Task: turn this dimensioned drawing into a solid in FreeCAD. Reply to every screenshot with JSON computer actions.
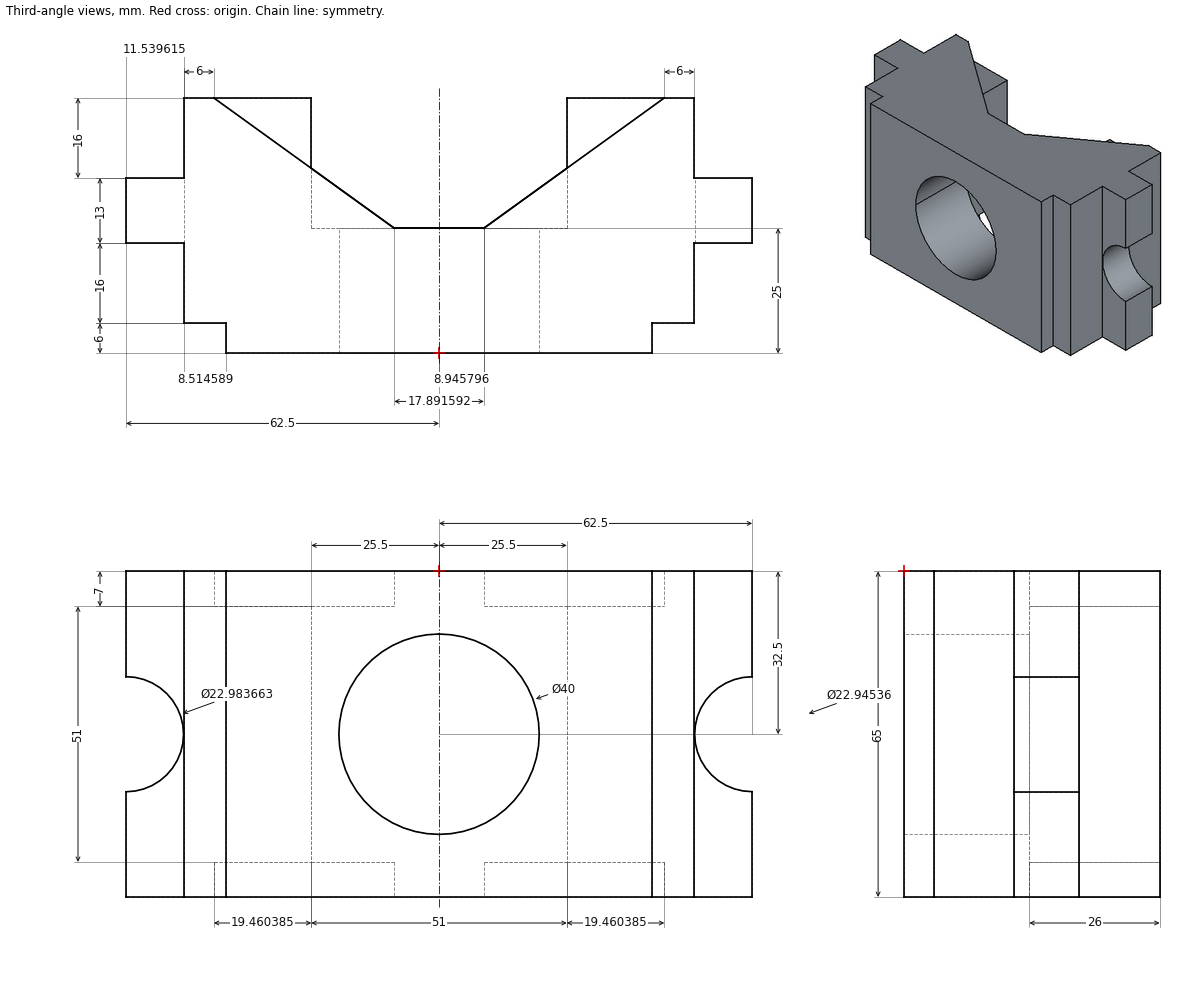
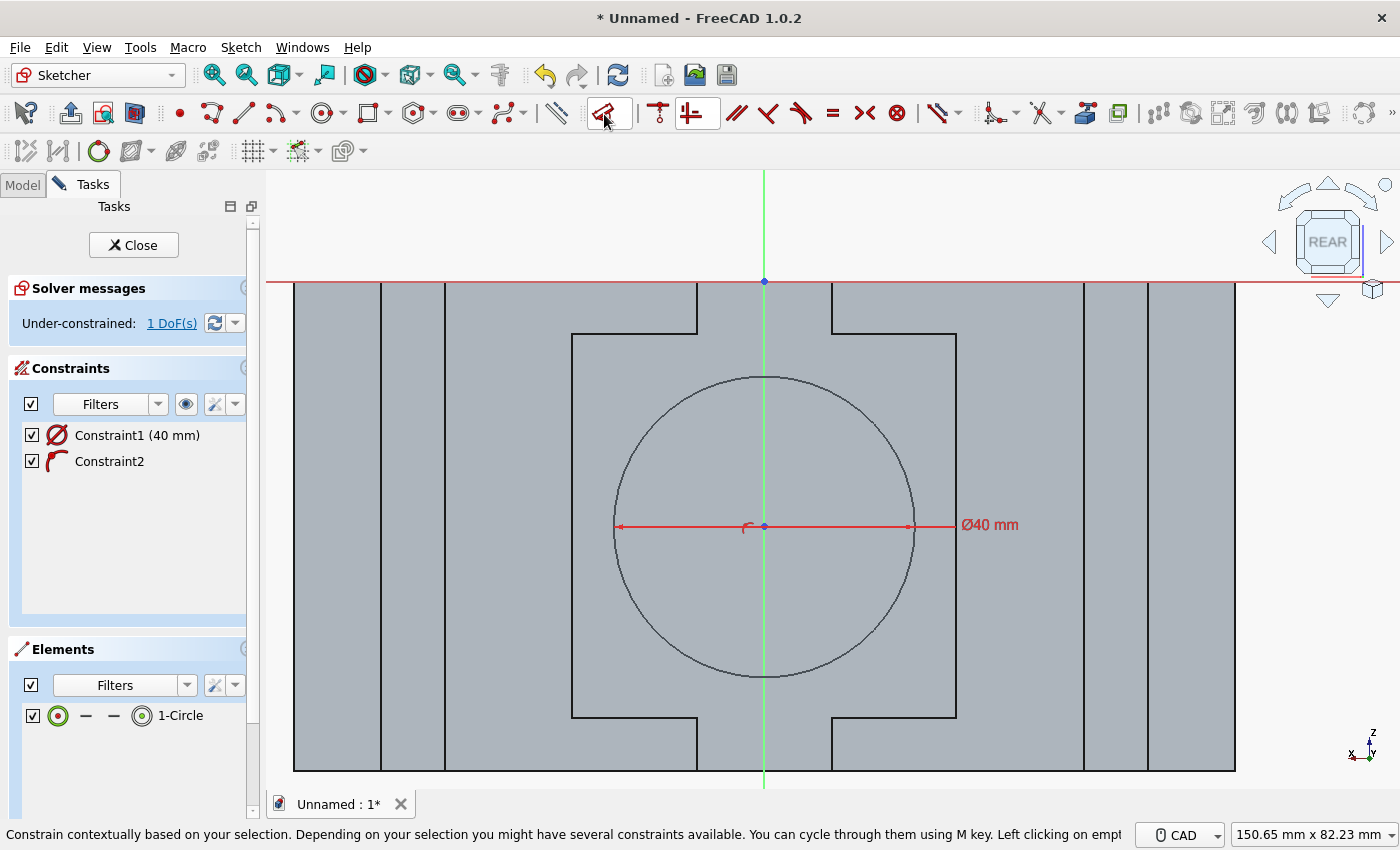
{"action": "left_click", "coordinate": [764, 527]}
{"action": "left_click", "coordinate": [798, 404]}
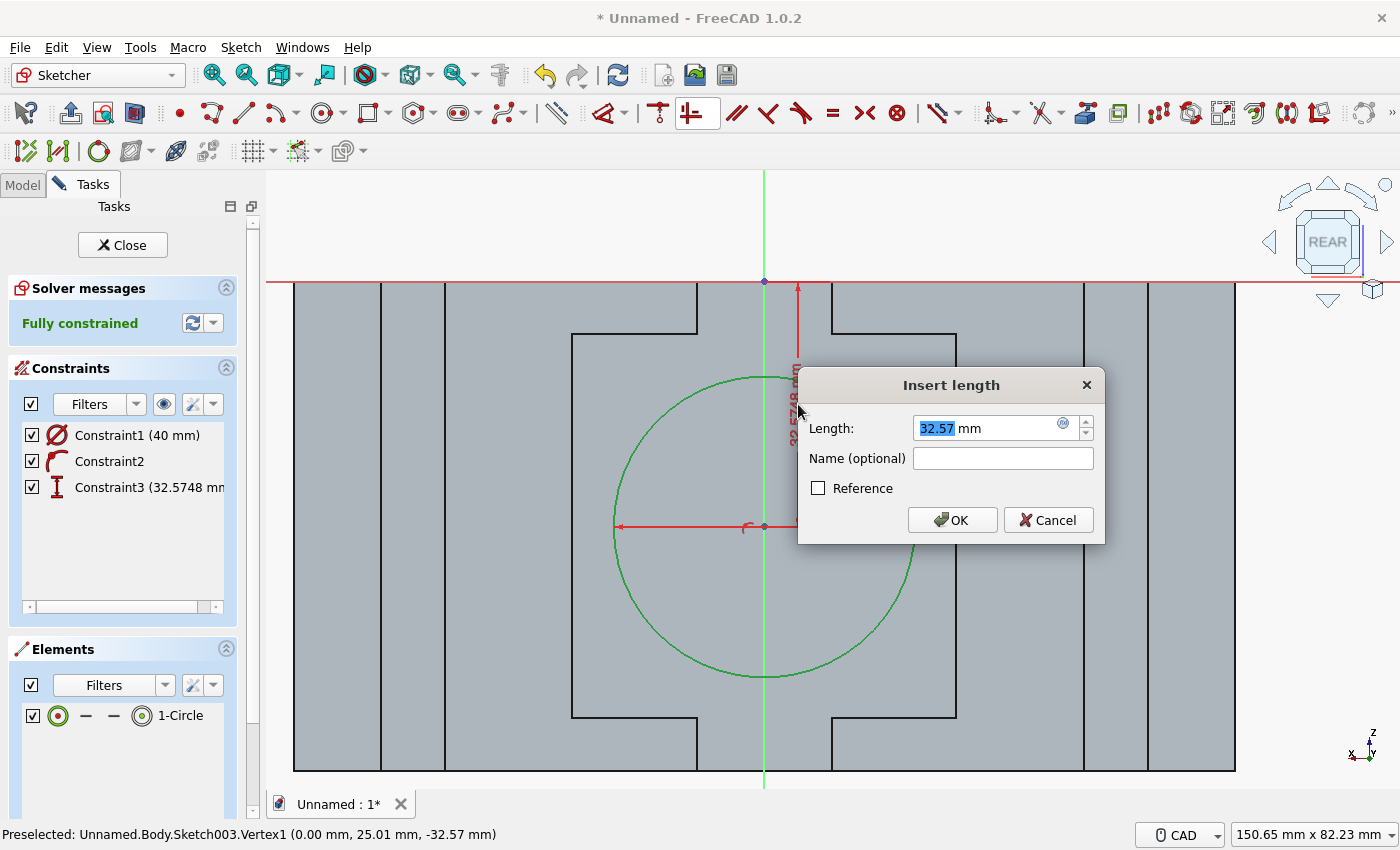
{"action": "type", "text": "32.5"}
{"action": "key", "text": "Return"}
{"action": "key", "text": "Escape"}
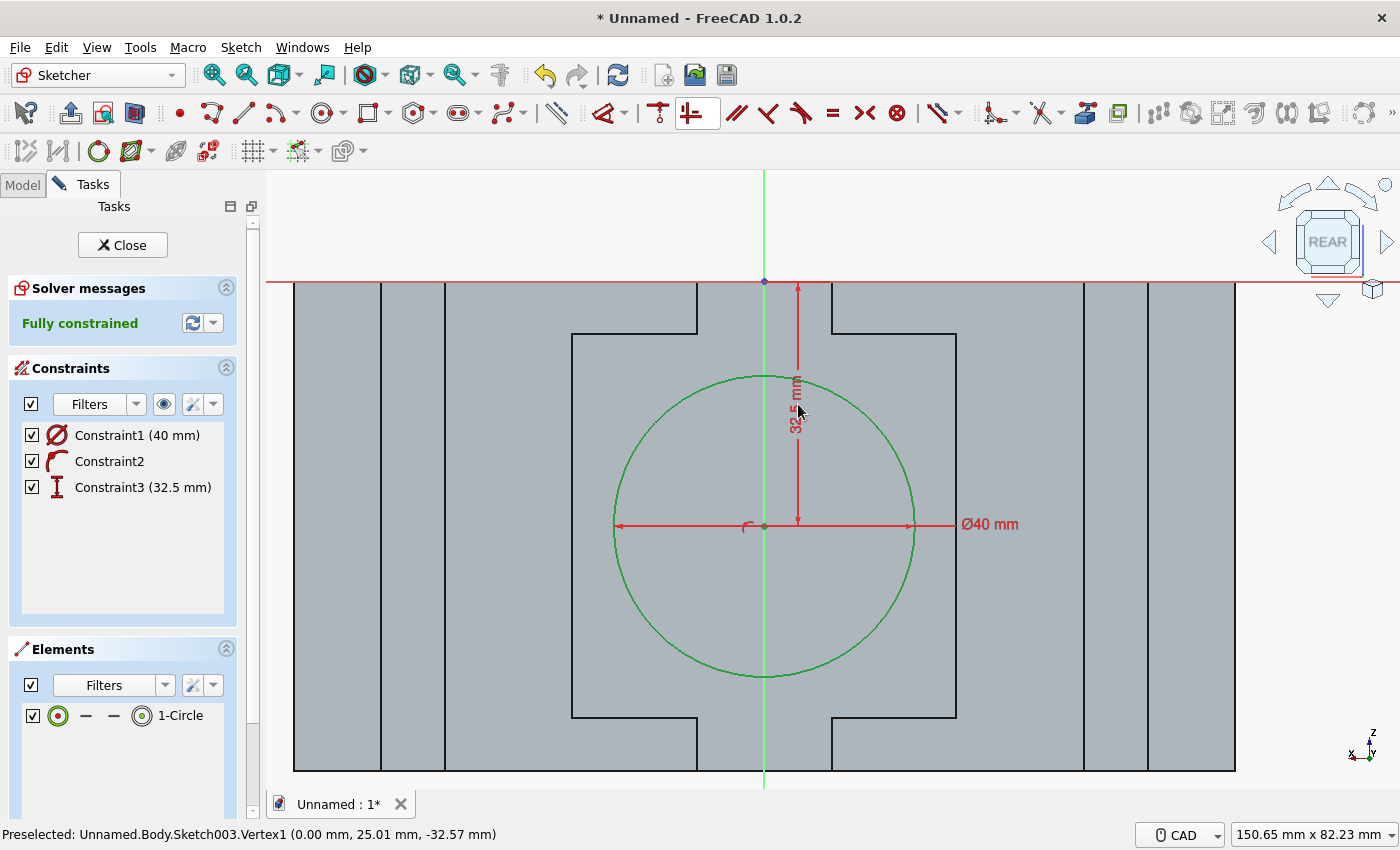
{"action": "left_click", "coordinate": [123, 245]}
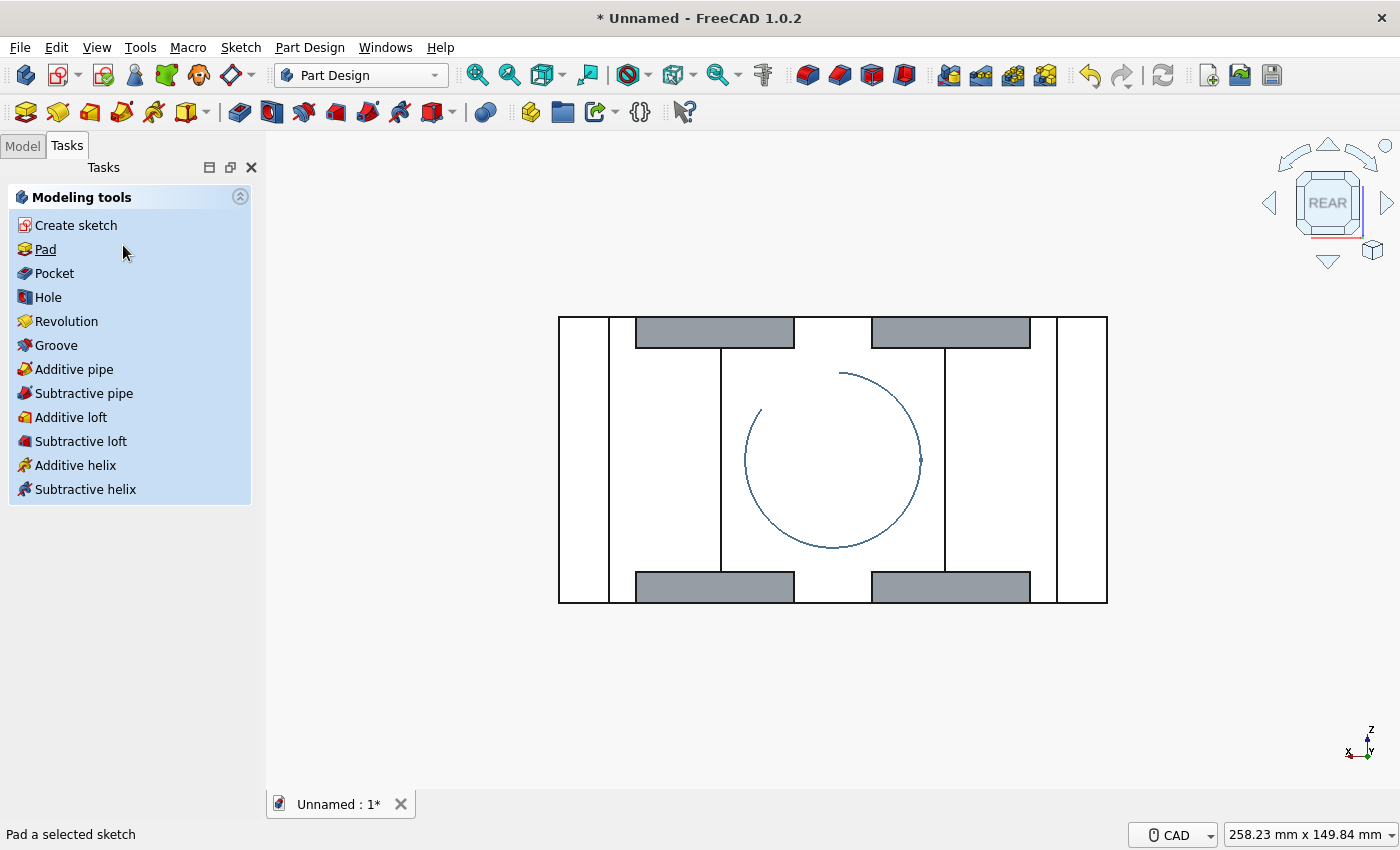
{"action": "left_click", "coordinate": [240, 112]}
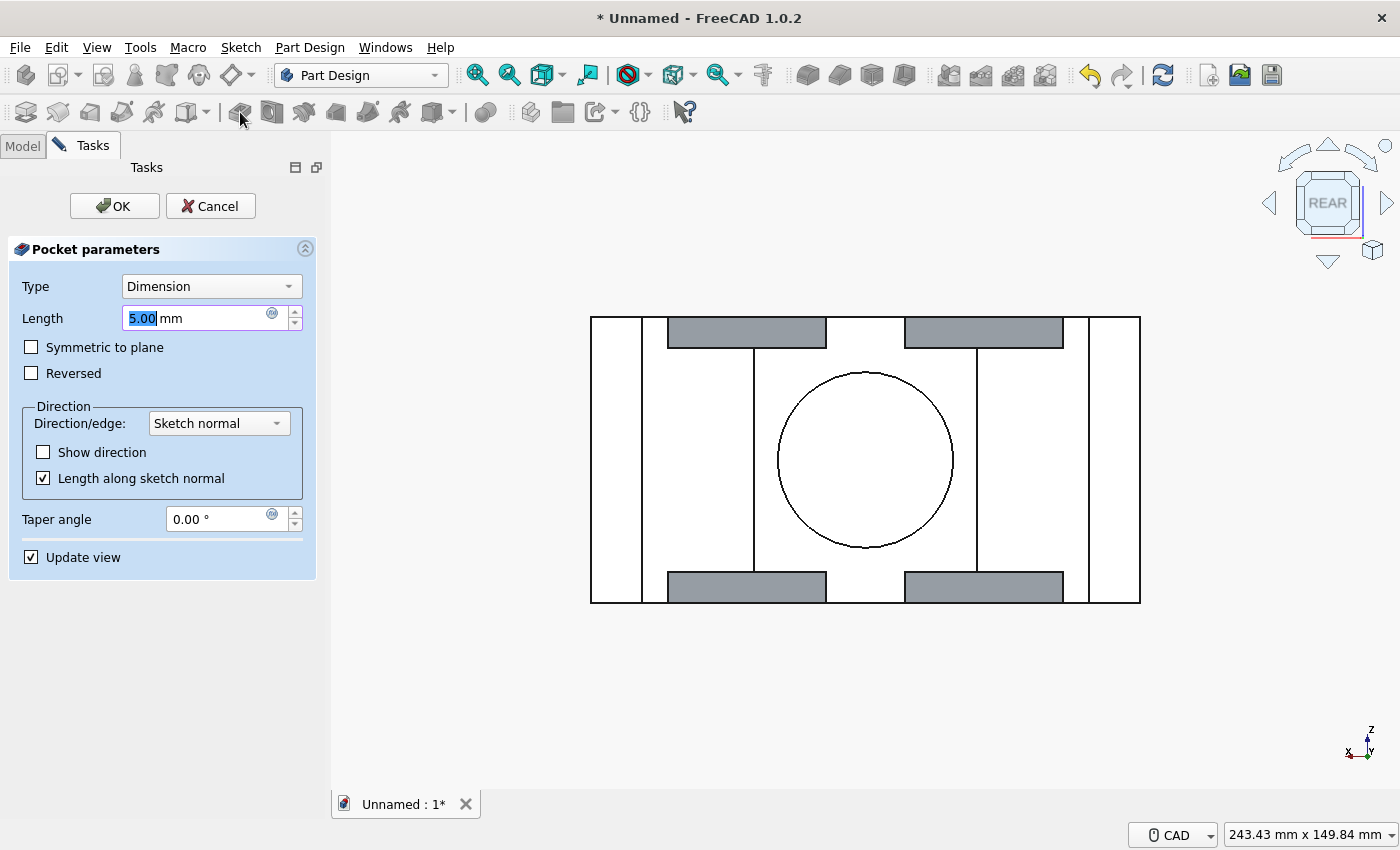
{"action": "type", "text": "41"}
{"action": "key", "text": "Tab"}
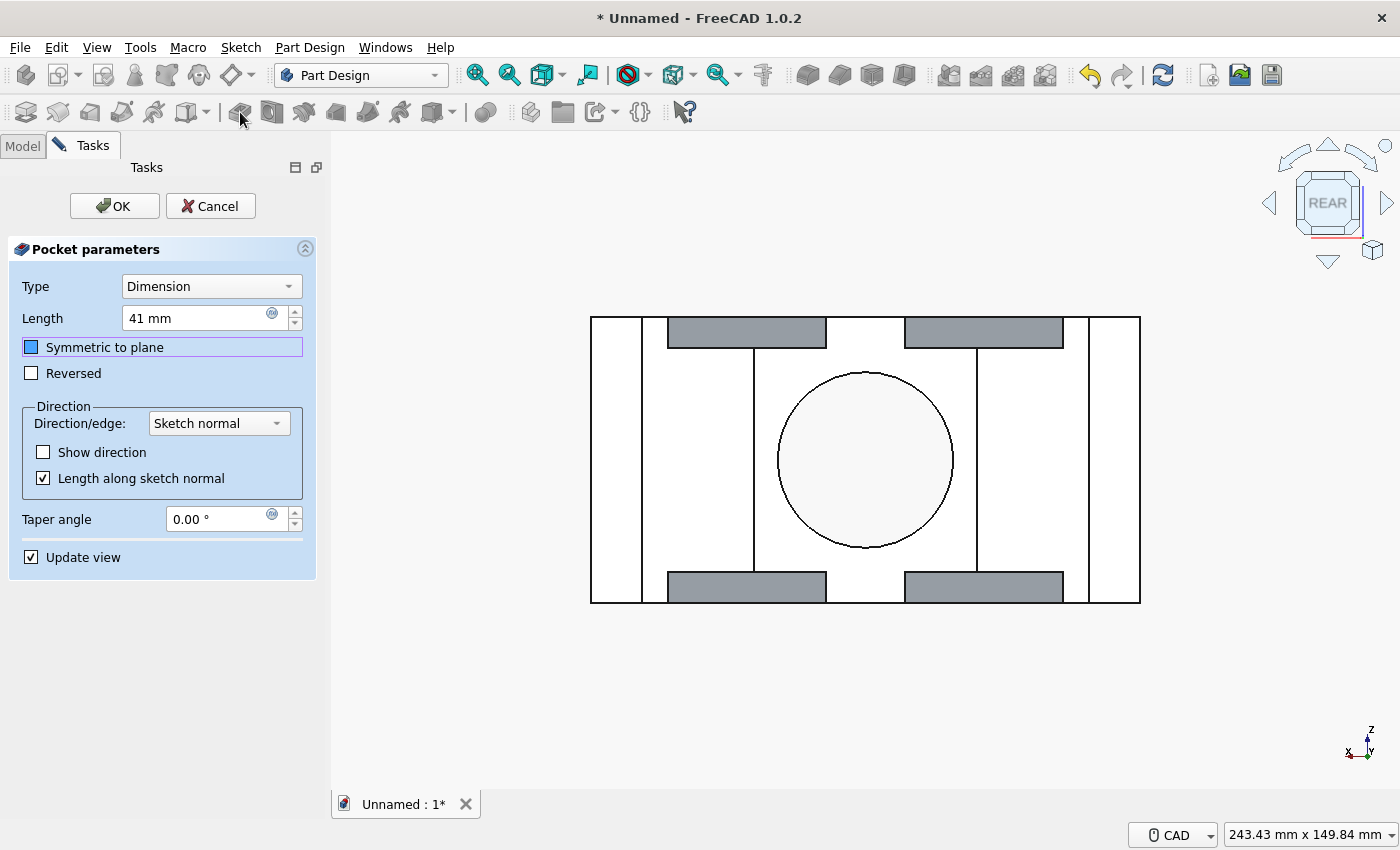
{"action": "left_click", "coordinate": [115, 206]}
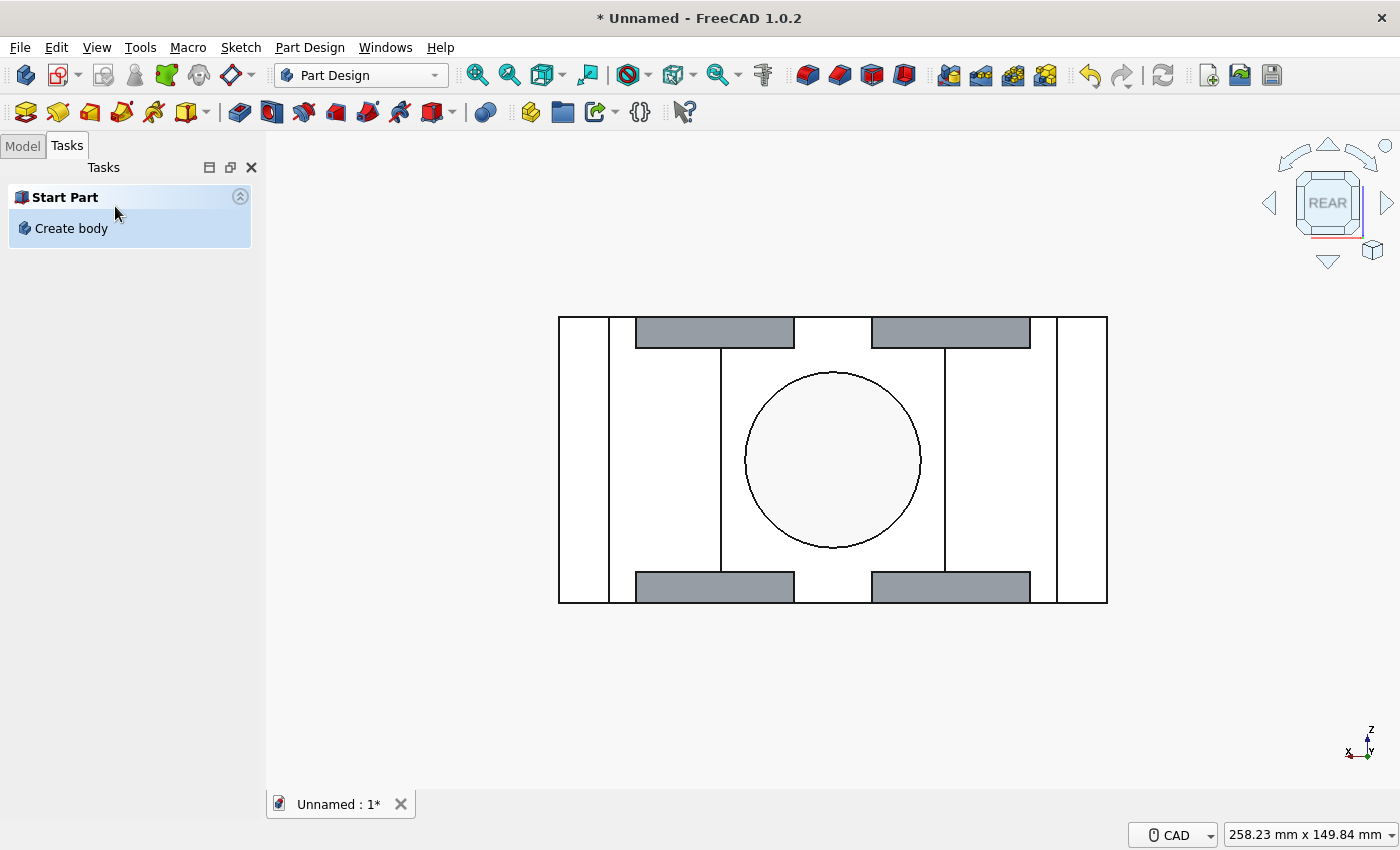
{"action": "left_click", "coordinate": [1082, 377]}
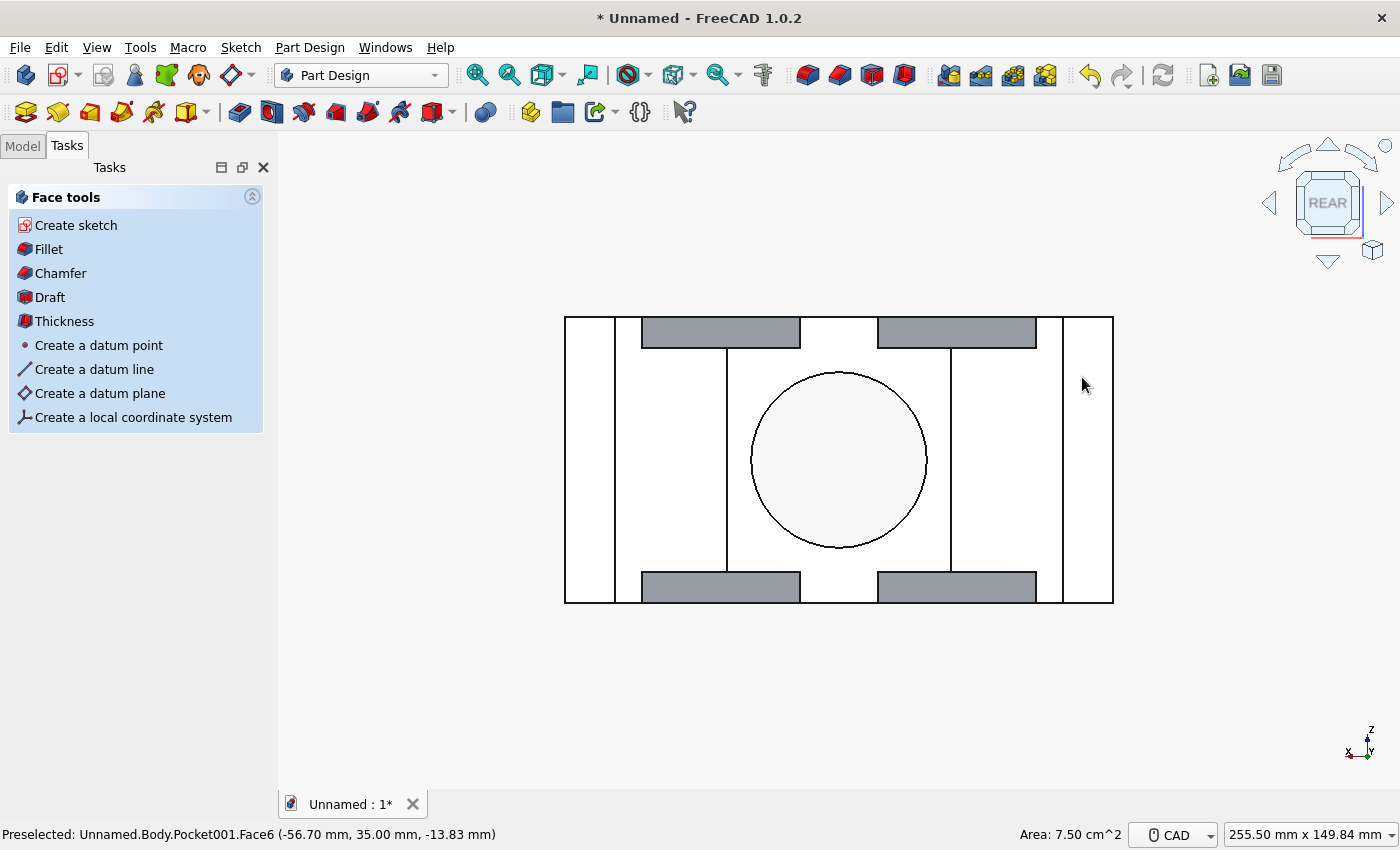
{"action": "left_click", "coordinate": [58, 76]}